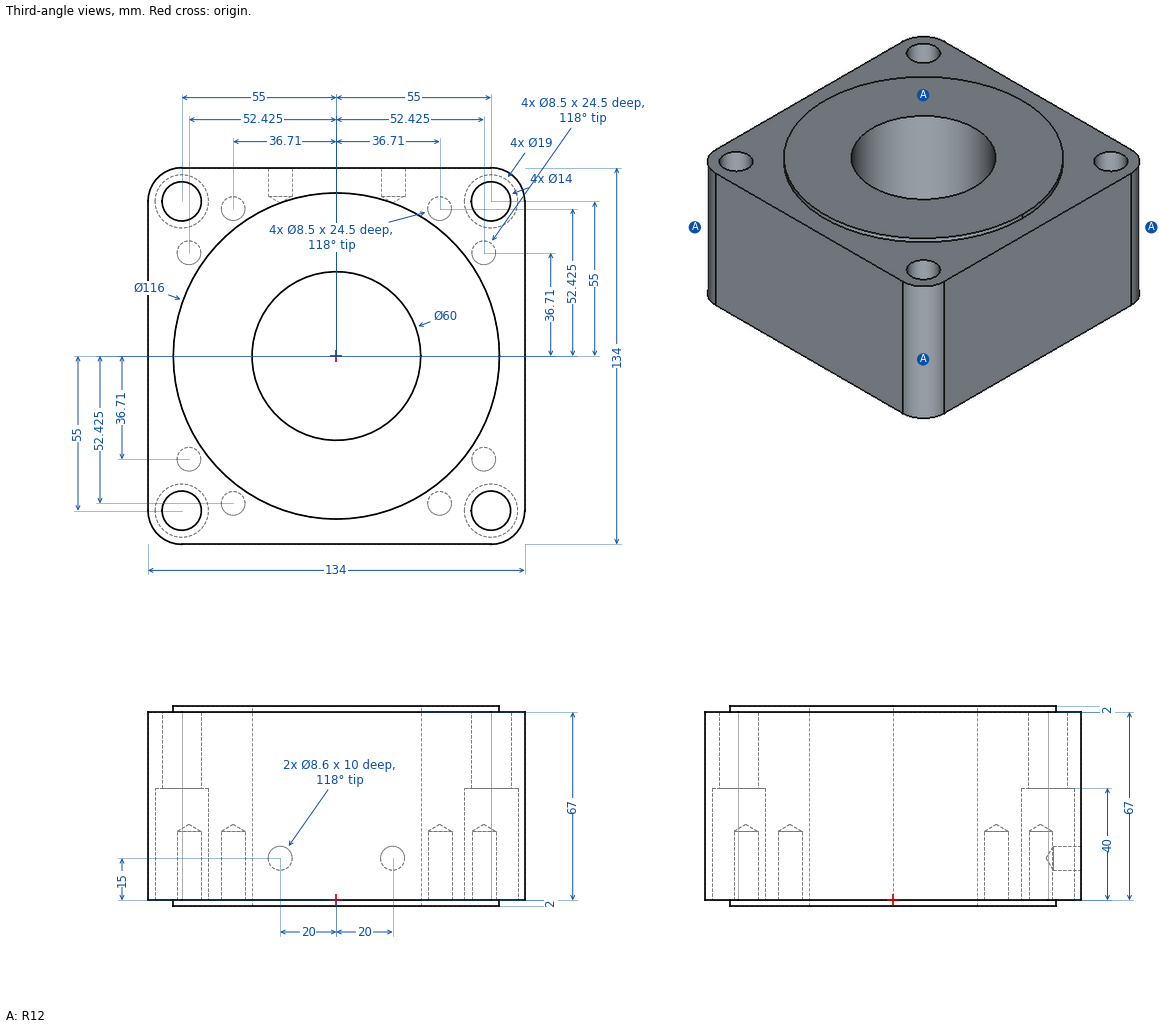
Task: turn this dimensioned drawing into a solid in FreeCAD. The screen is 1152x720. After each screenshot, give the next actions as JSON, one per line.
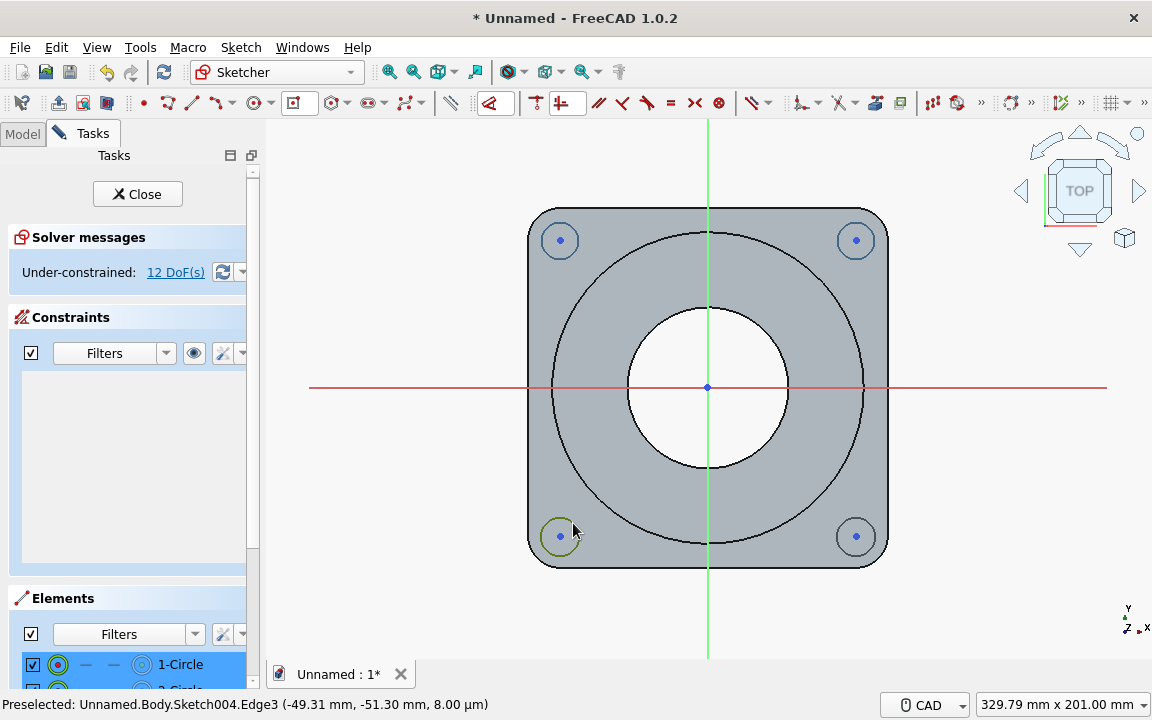
{"action": "left_click", "coordinate": [869, 523]}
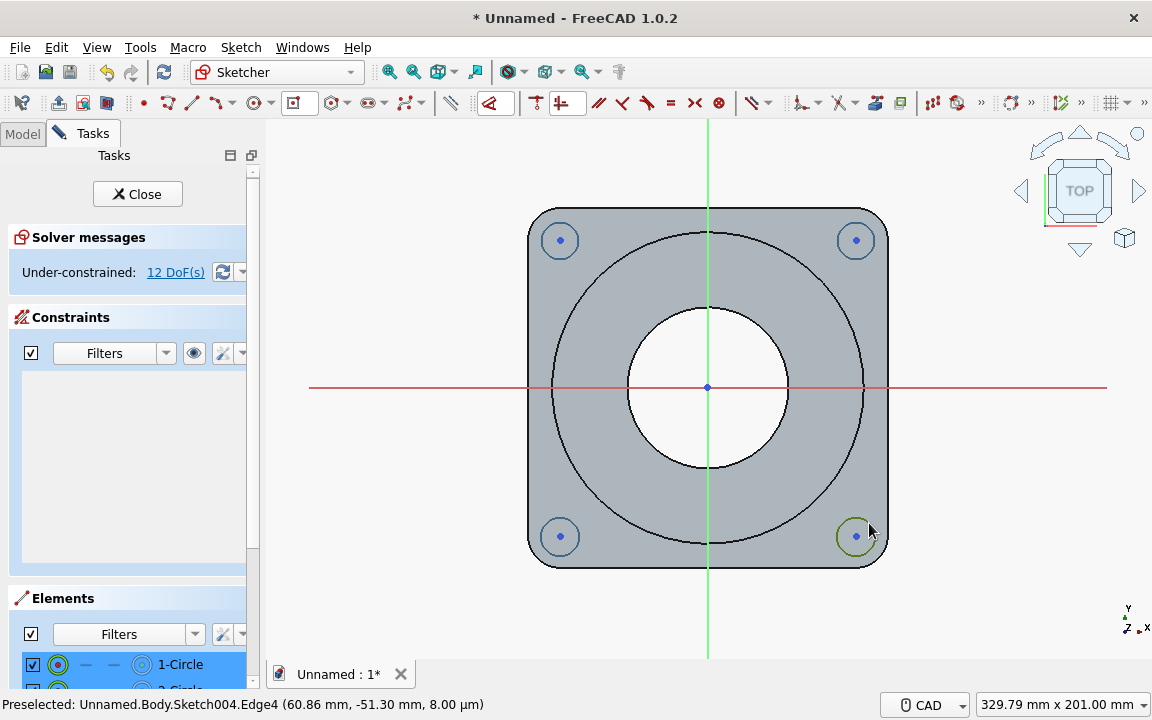
{"action": "left_click", "coordinate": [672, 104]}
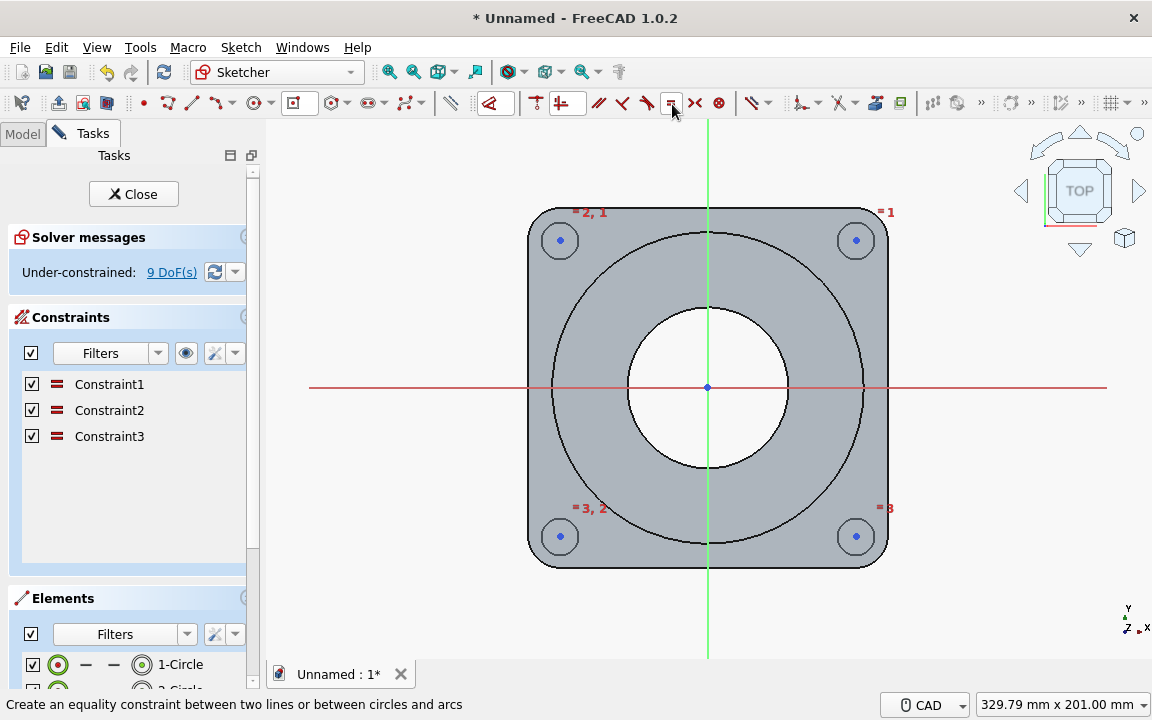
{"action": "left_click", "coordinate": [856, 241]}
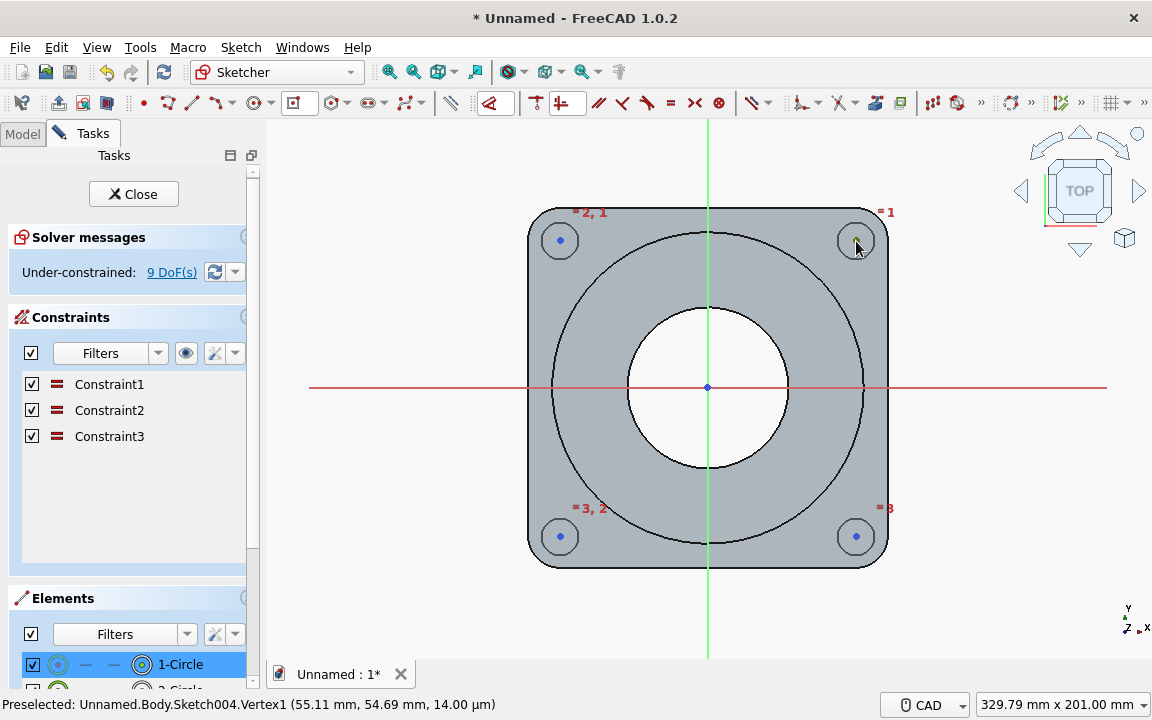
{"action": "left_click", "coordinate": [560, 241]}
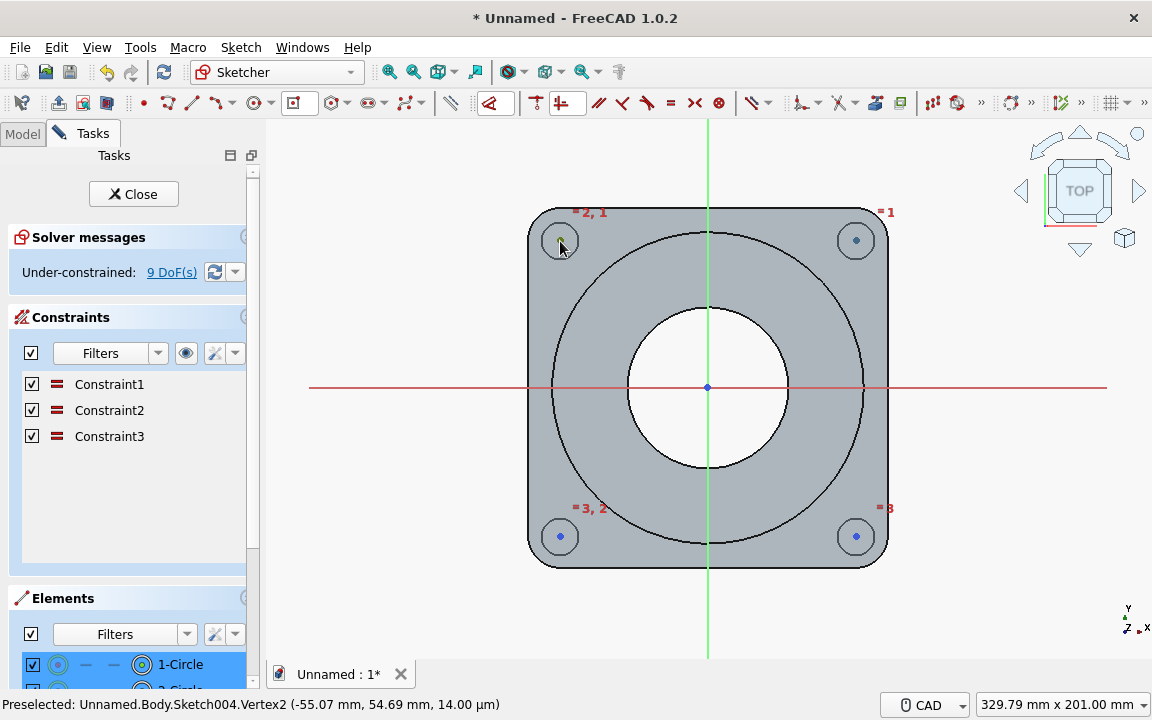
{"action": "key", "text": "h"}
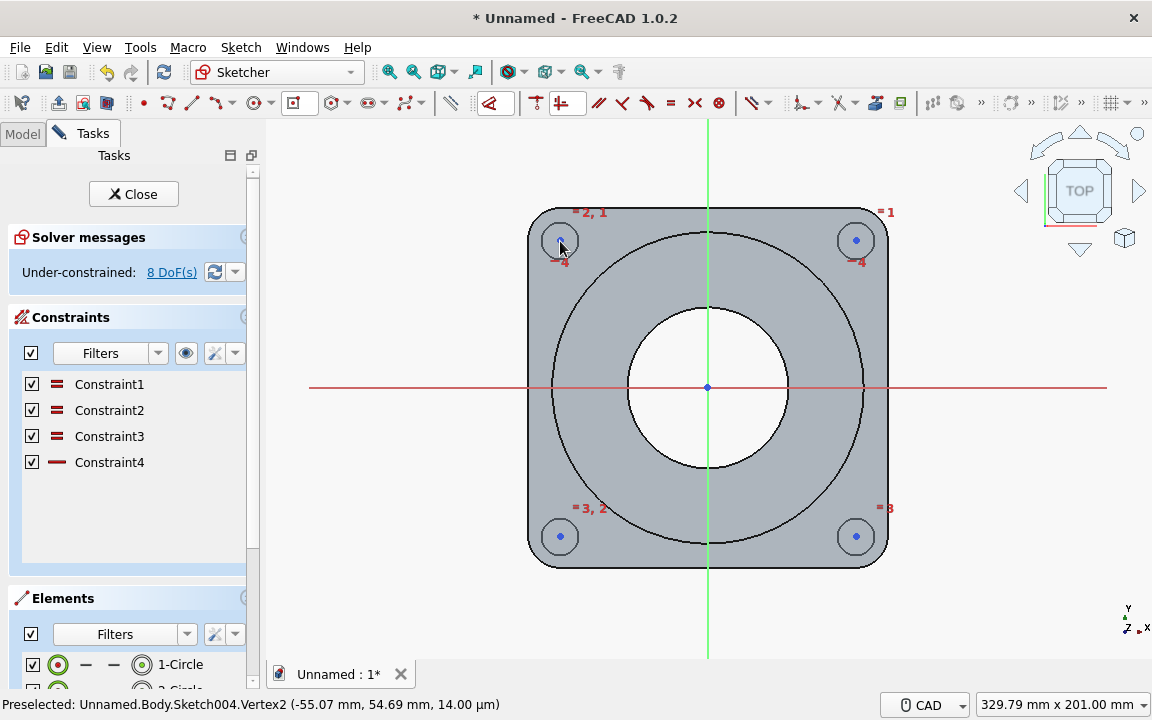
{"action": "left_click", "coordinate": [560, 241]}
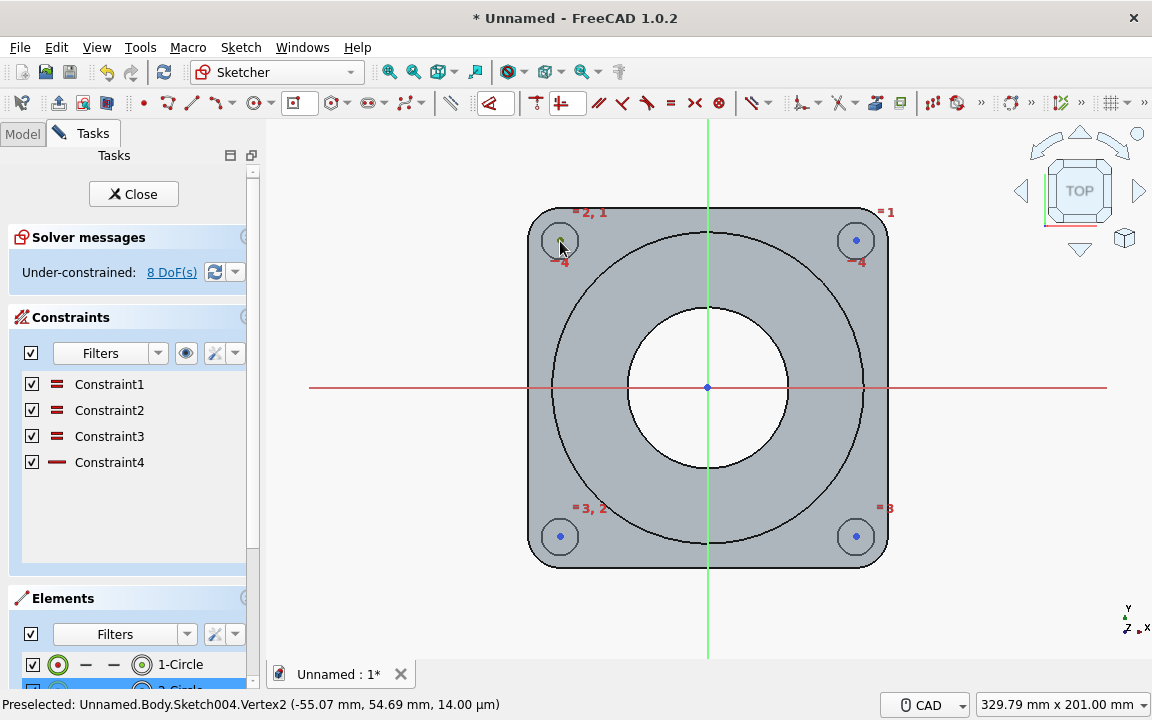
{"action": "left_click", "coordinate": [560, 537]}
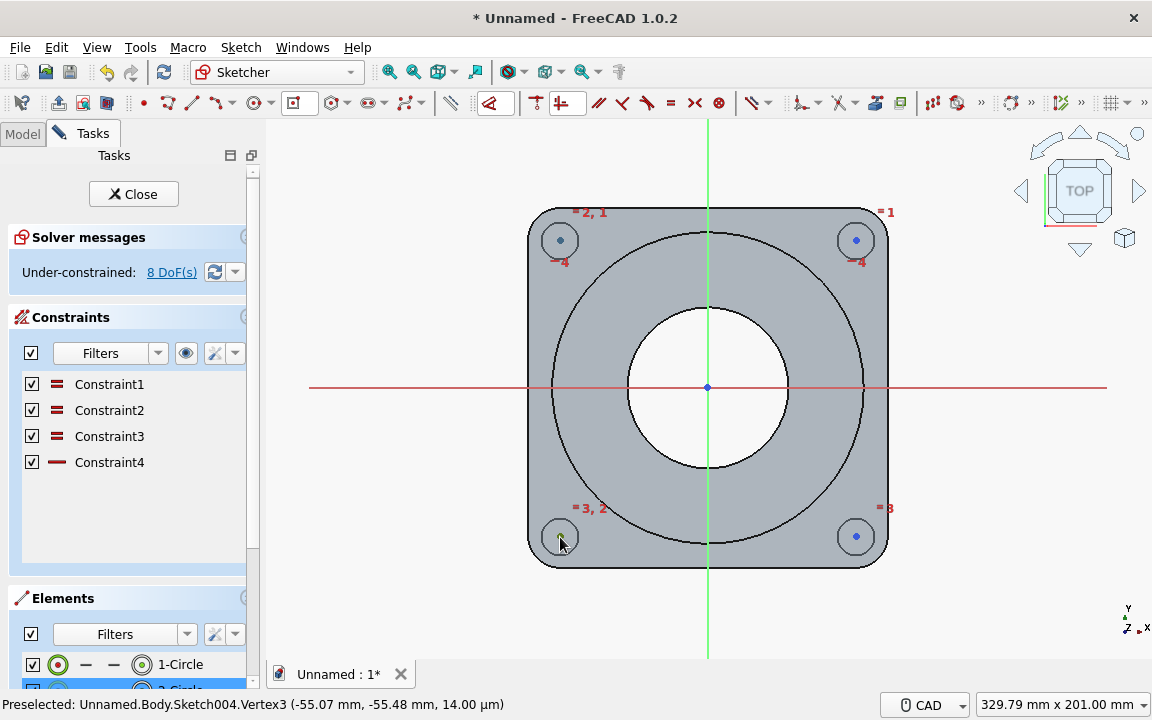
{"action": "key", "text": "v"}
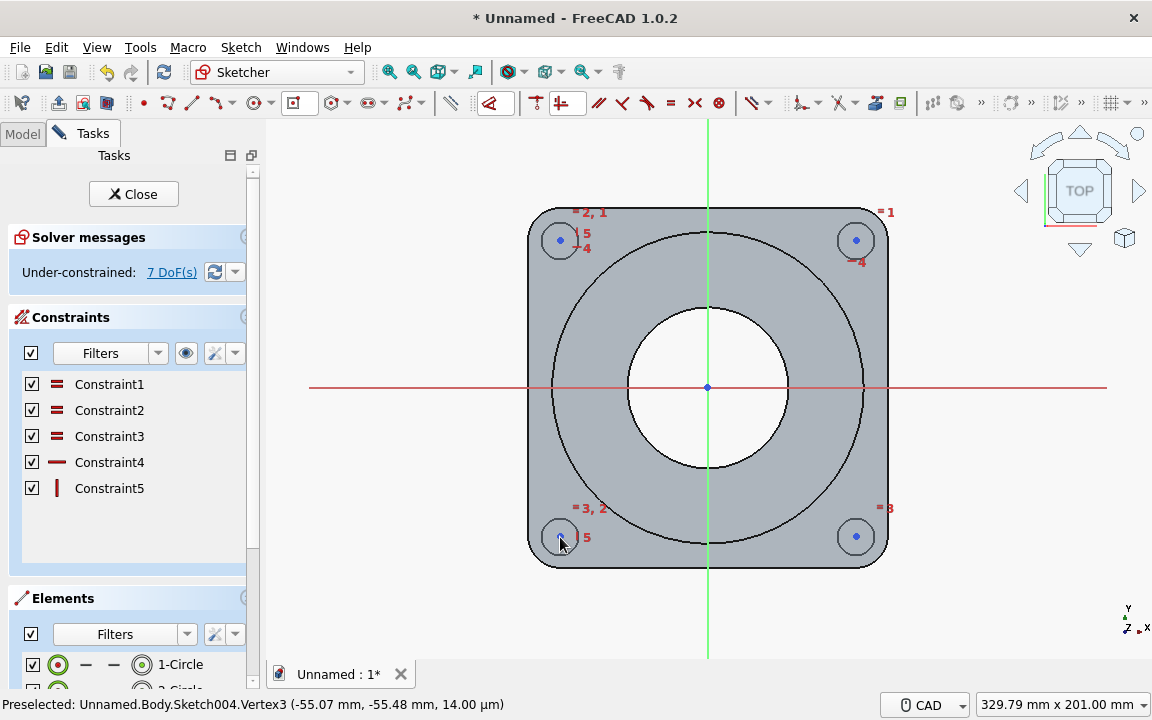
{"action": "left_click", "coordinate": [856, 241]}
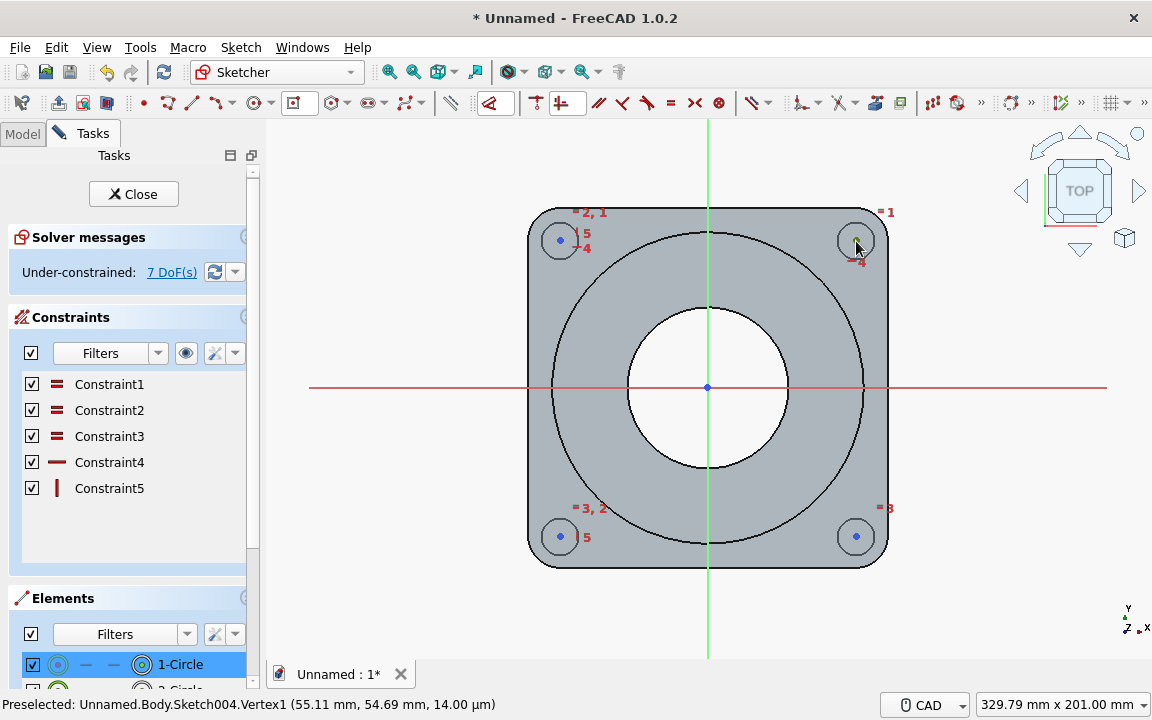
{"action": "left_click", "coordinate": [856, 537]}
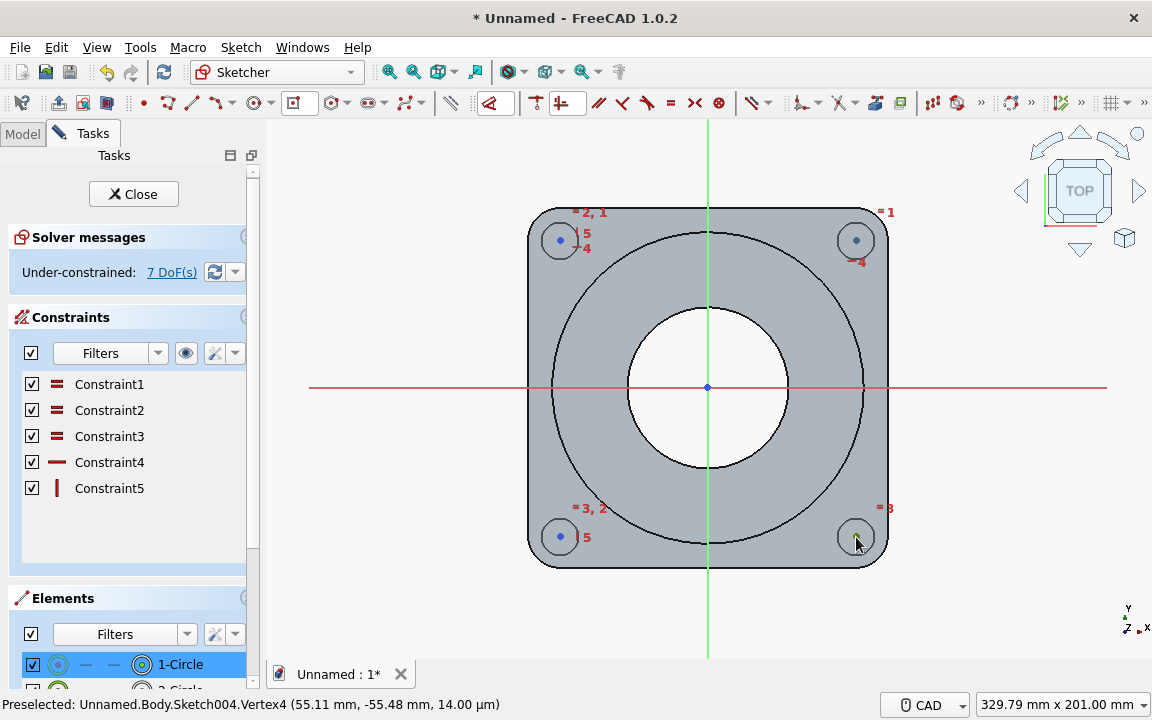
{"action": "left_click", "coordinate": [580, 104]}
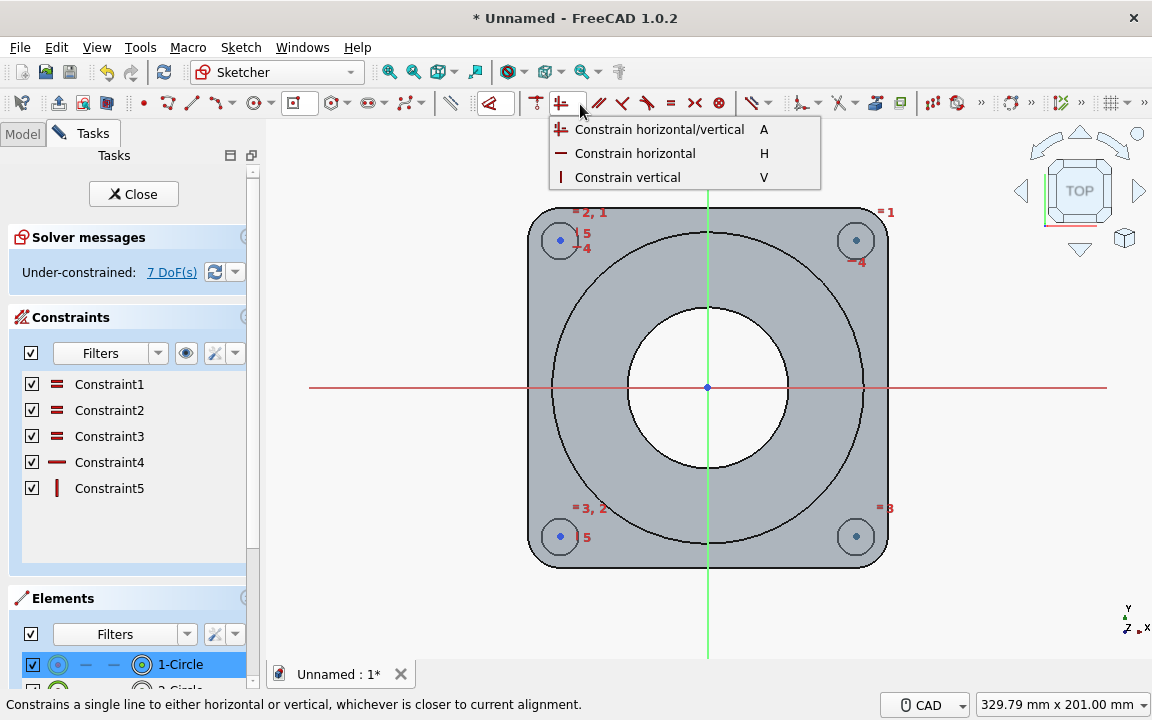
{"action": "left_click", "coordinate": [685, 177]}